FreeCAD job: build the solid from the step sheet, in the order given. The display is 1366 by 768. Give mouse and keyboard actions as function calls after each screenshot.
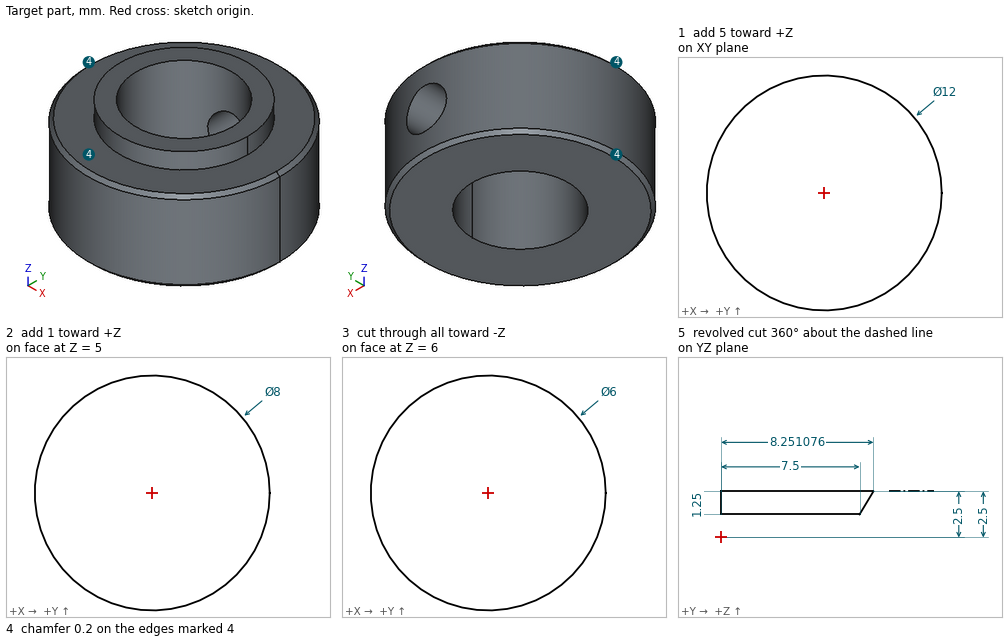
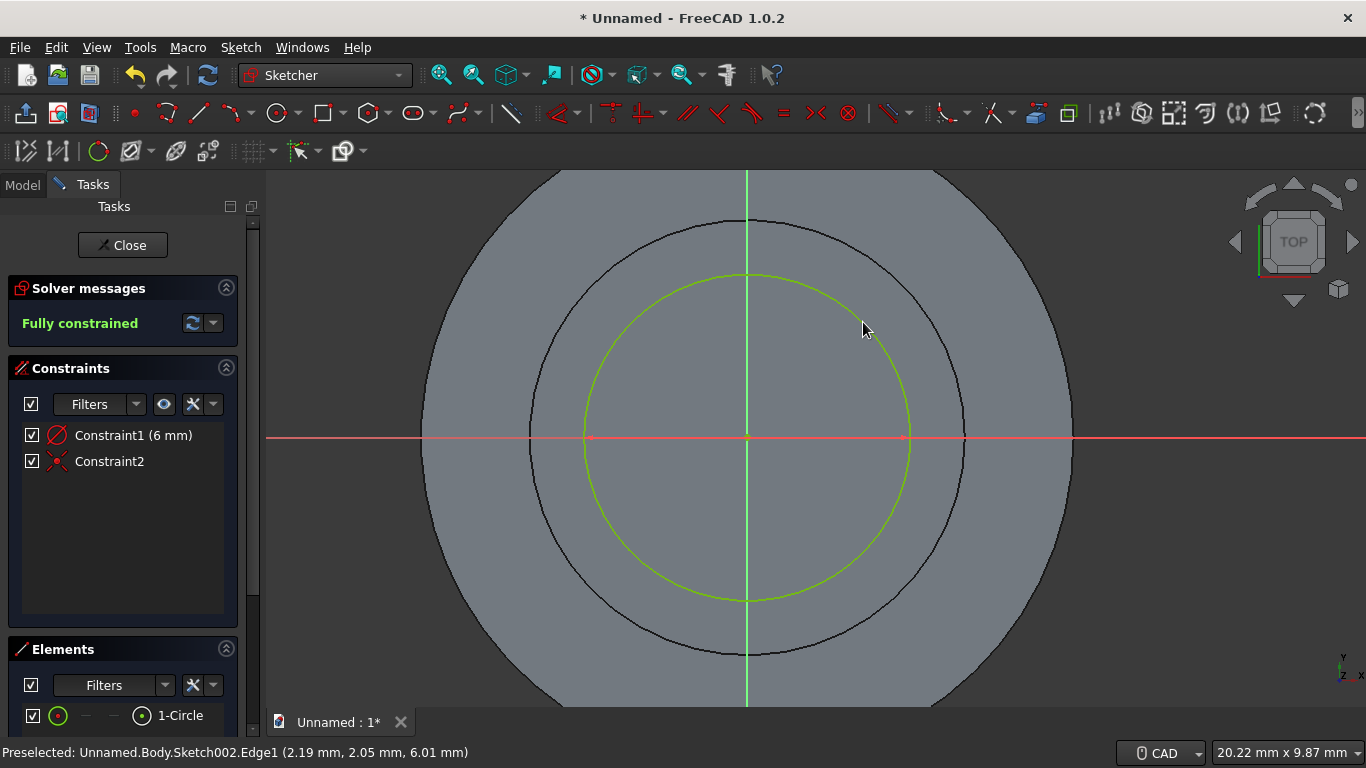
click(123, 245)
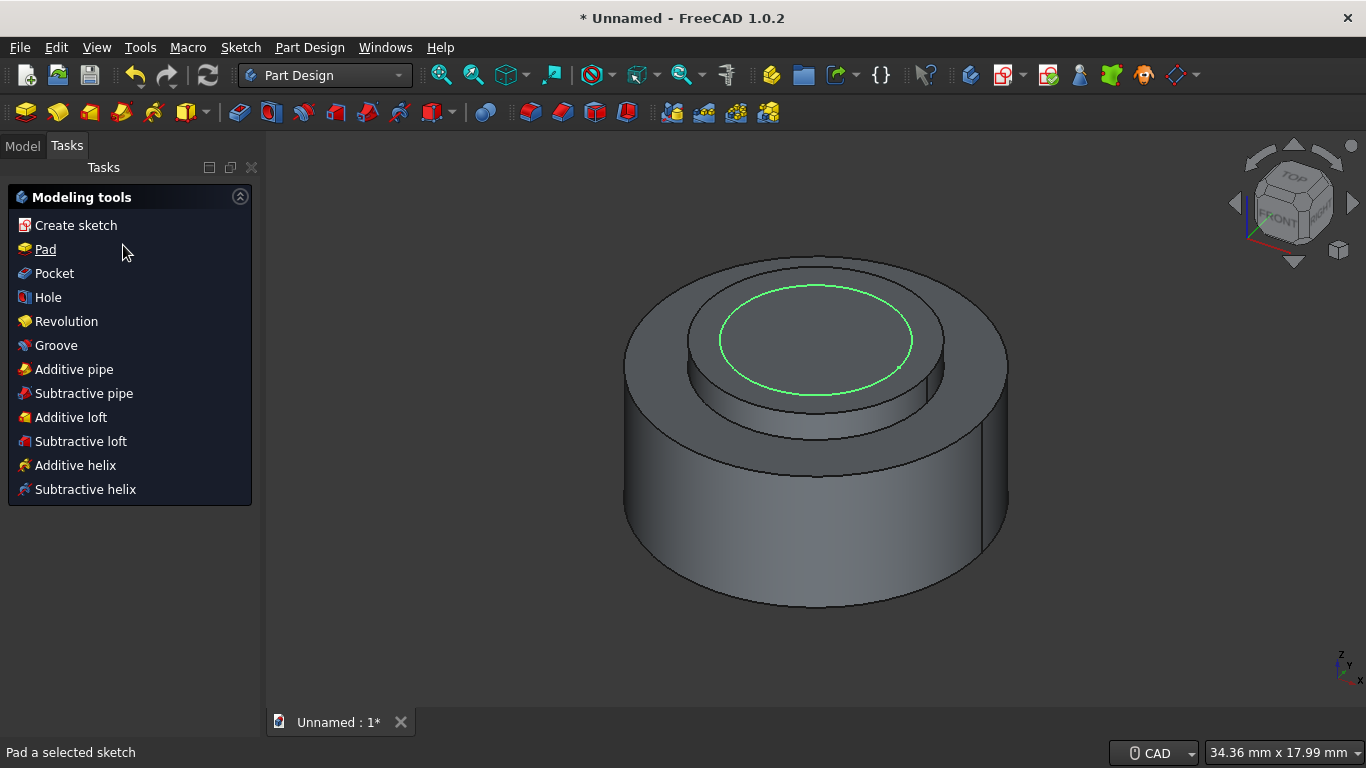
click(240, 112)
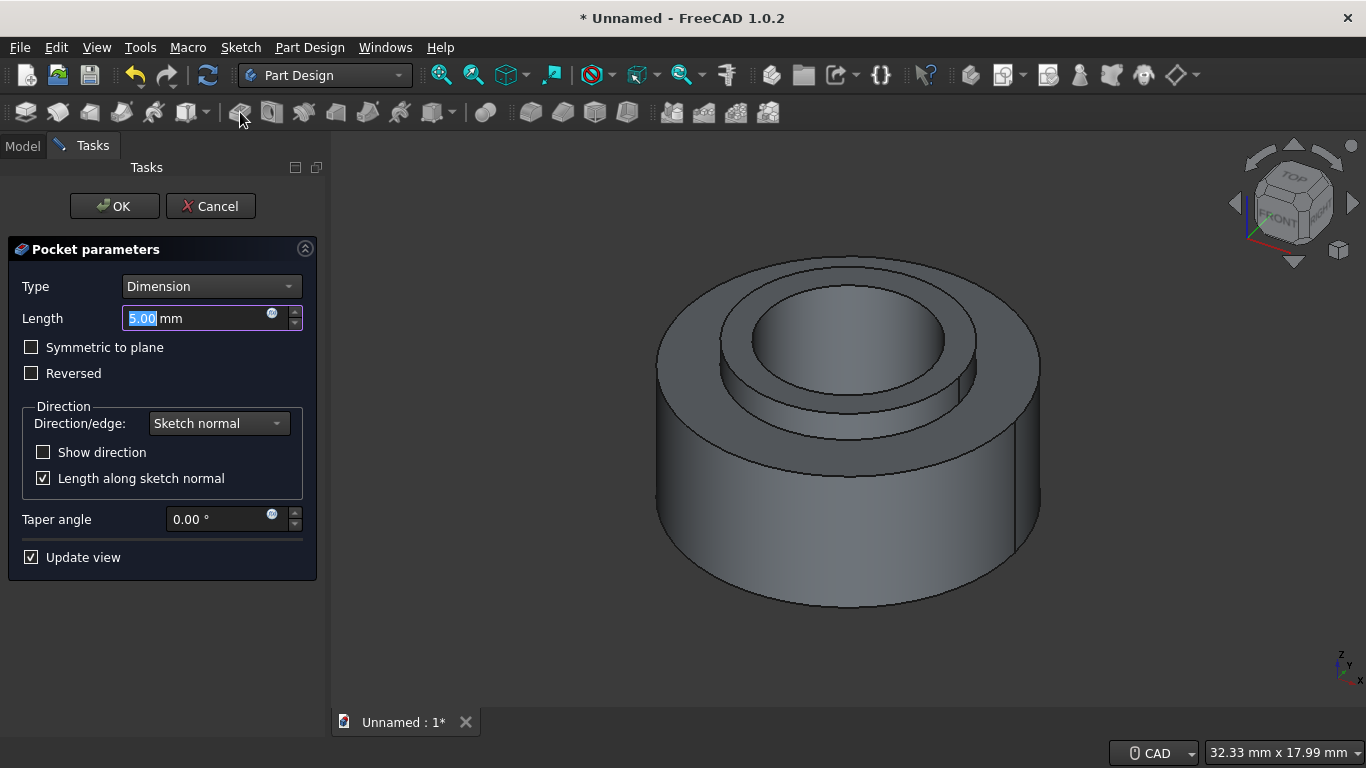
click(212, 286)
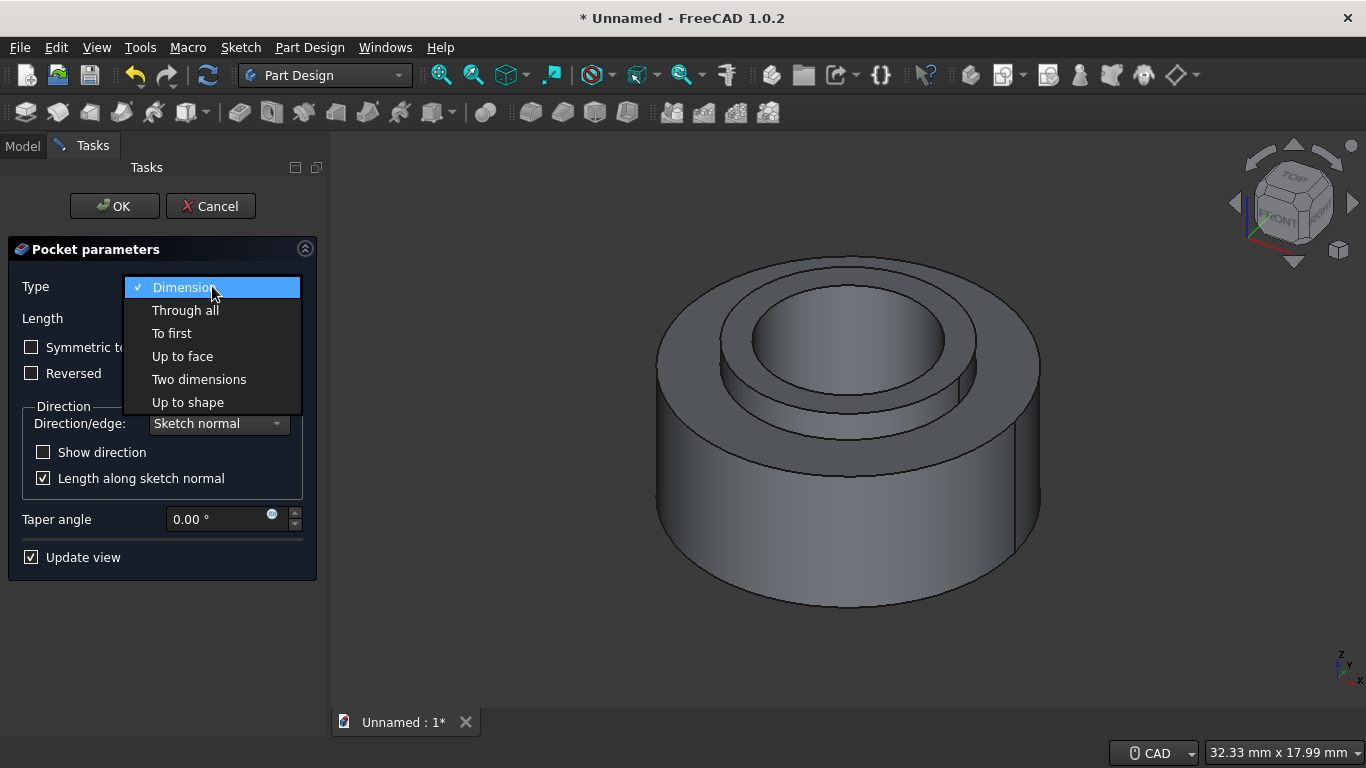
click(212, 310)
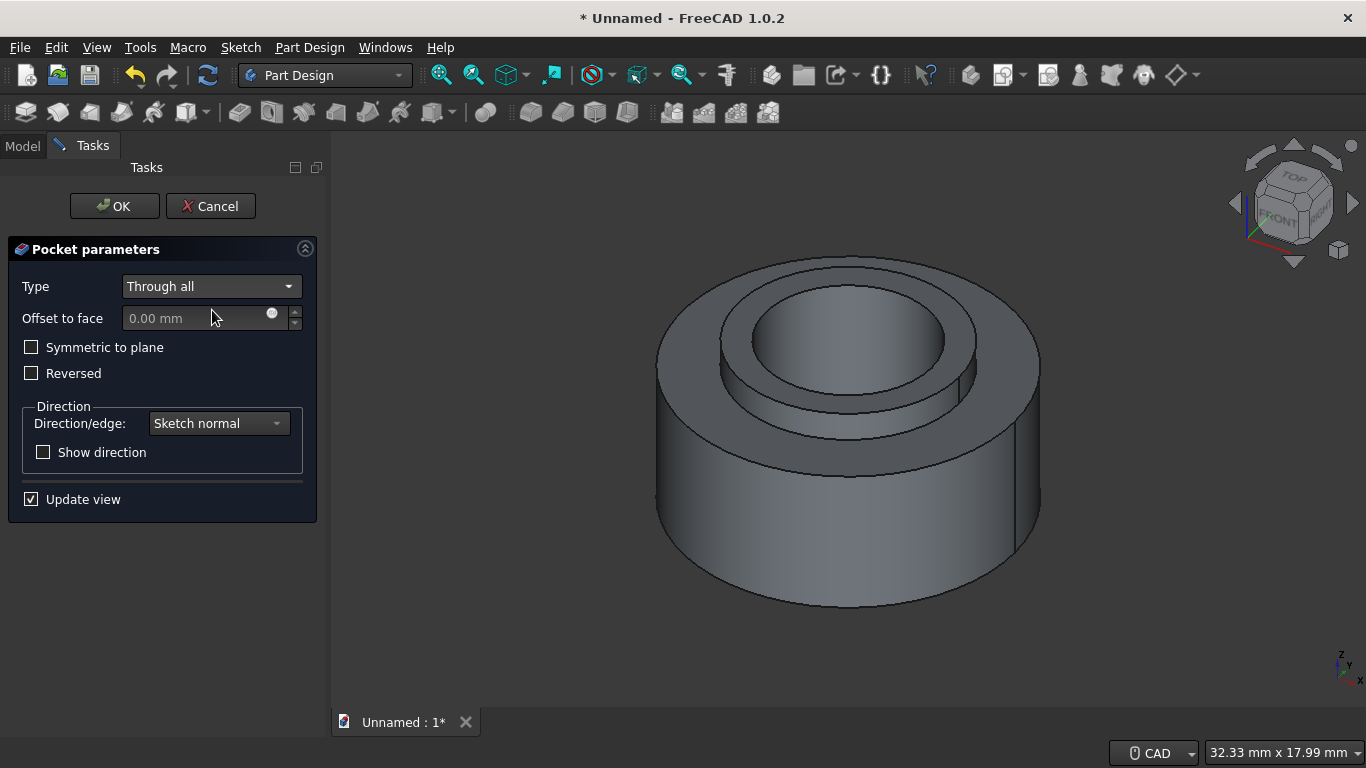
click(115, 206)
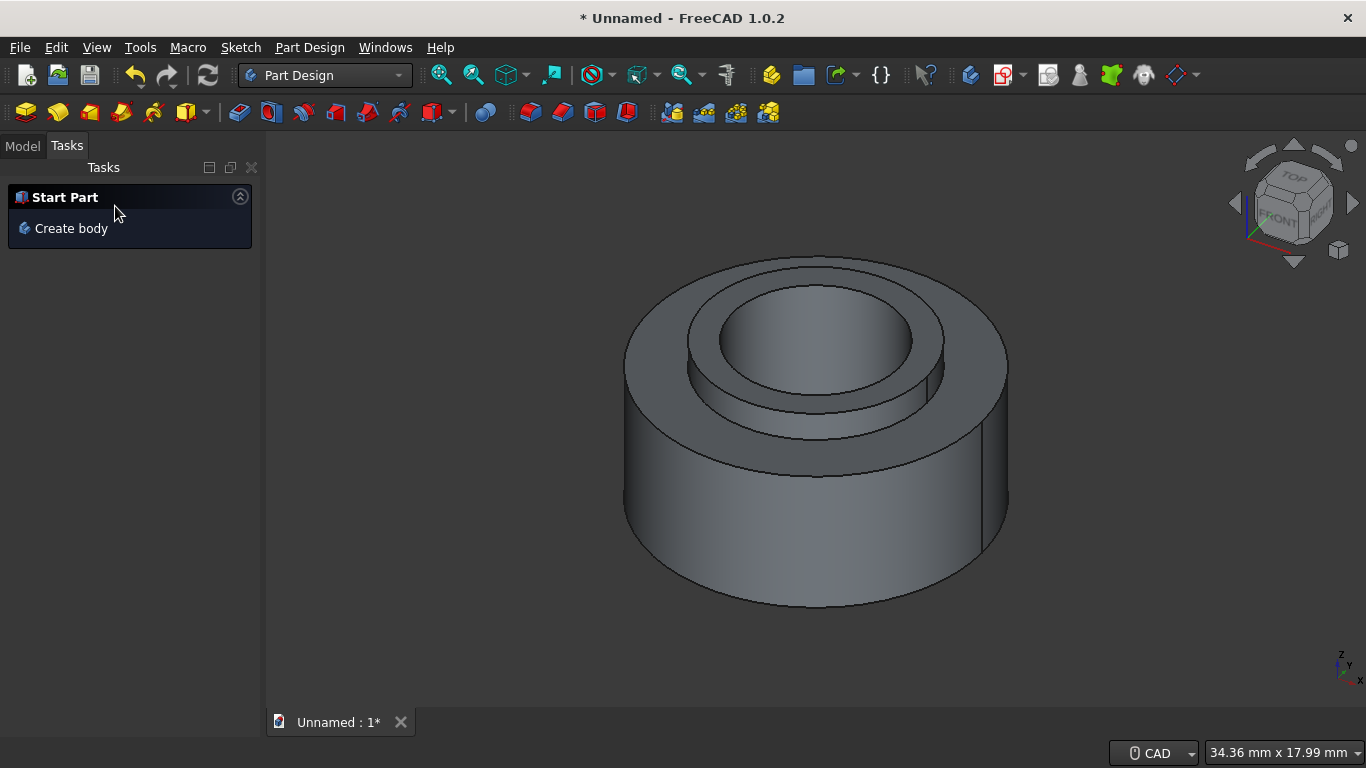
click(625, 377)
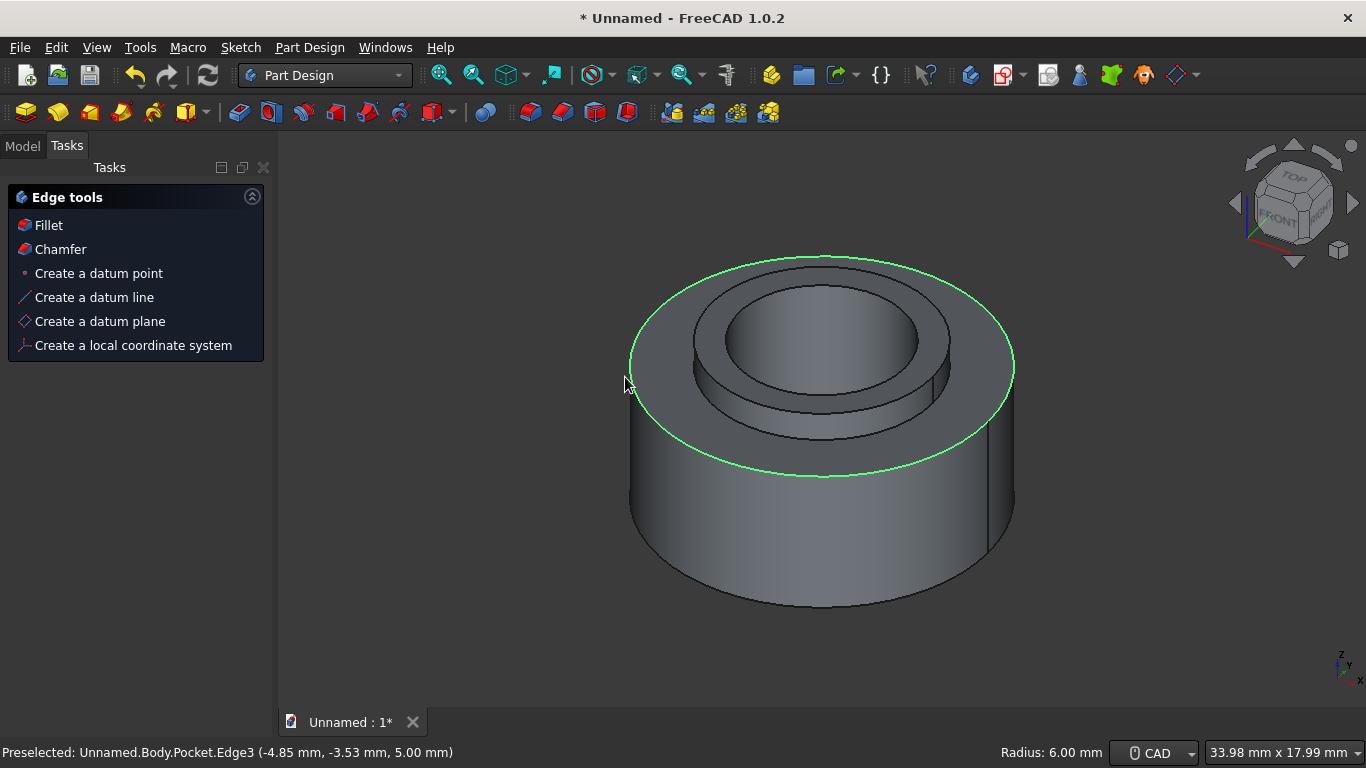
key(0)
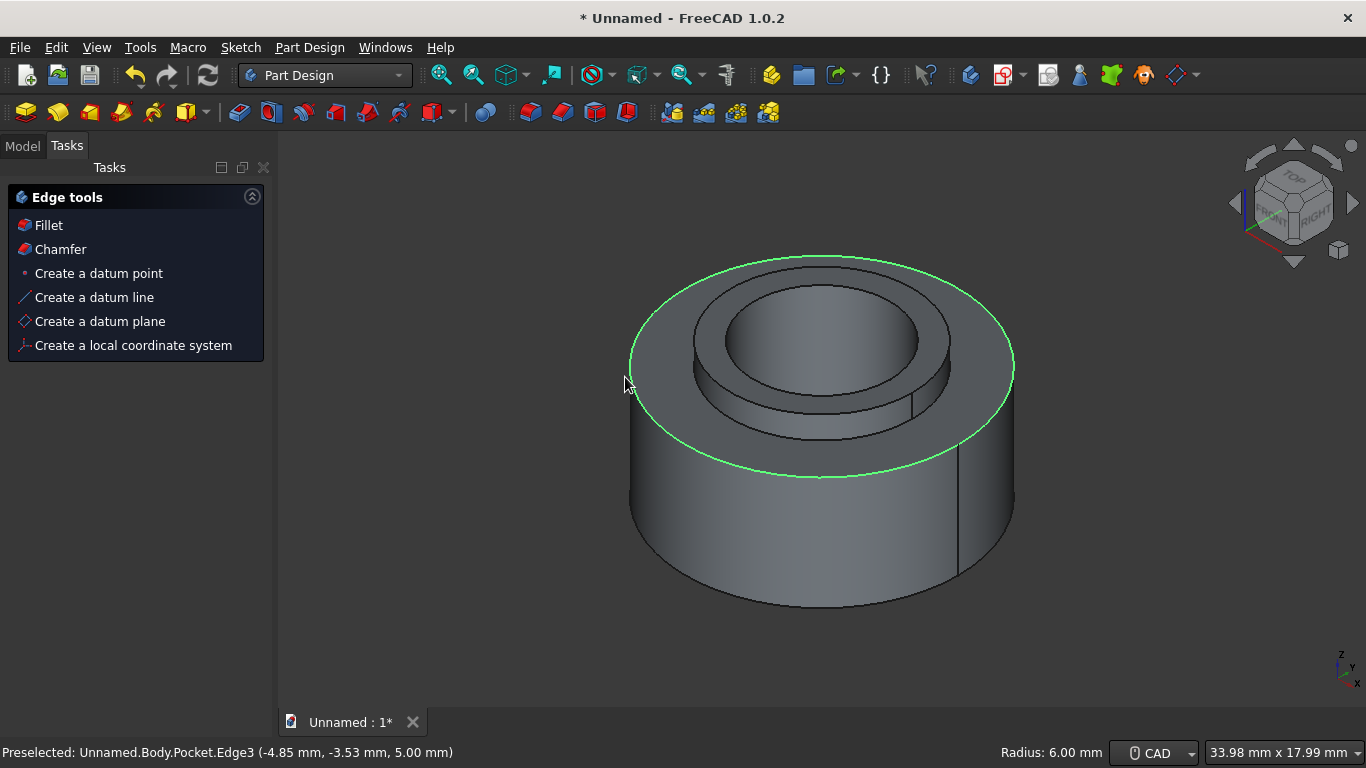
key(2)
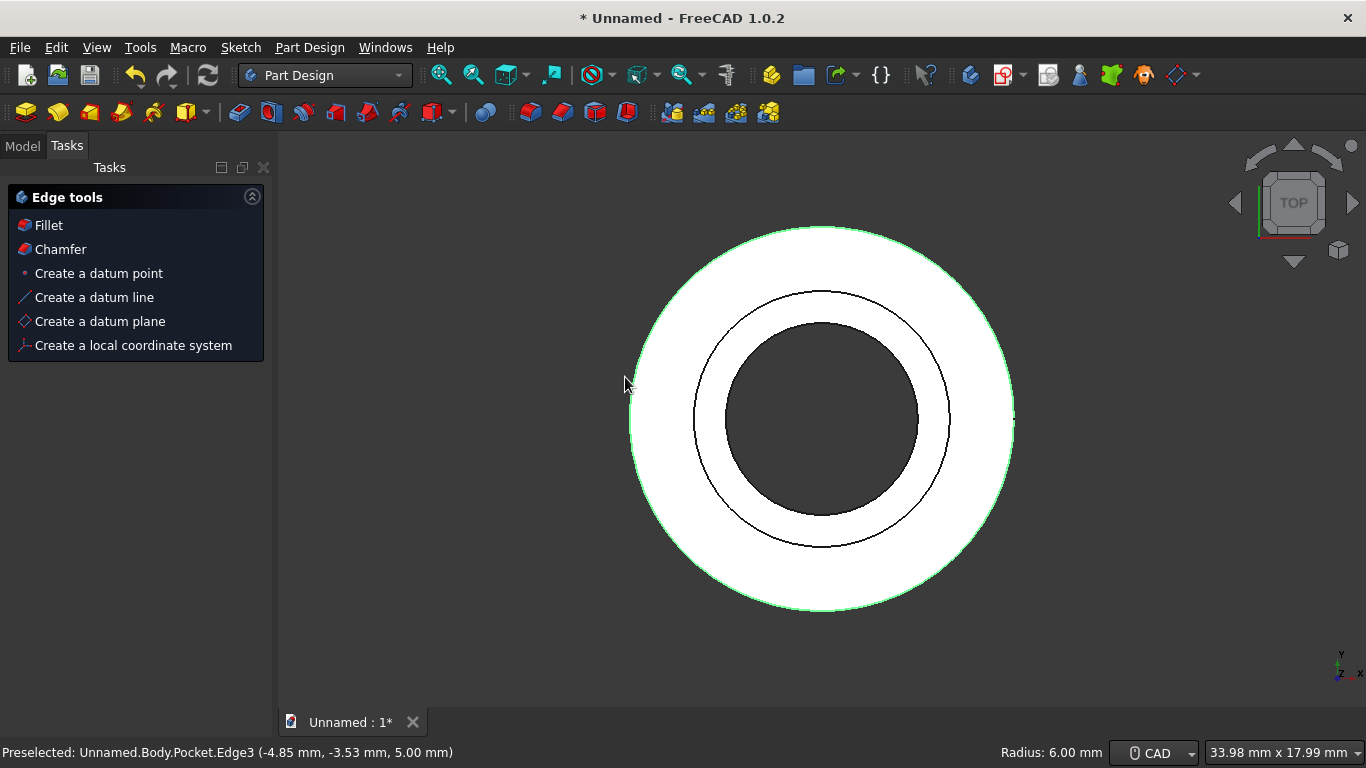
key(1)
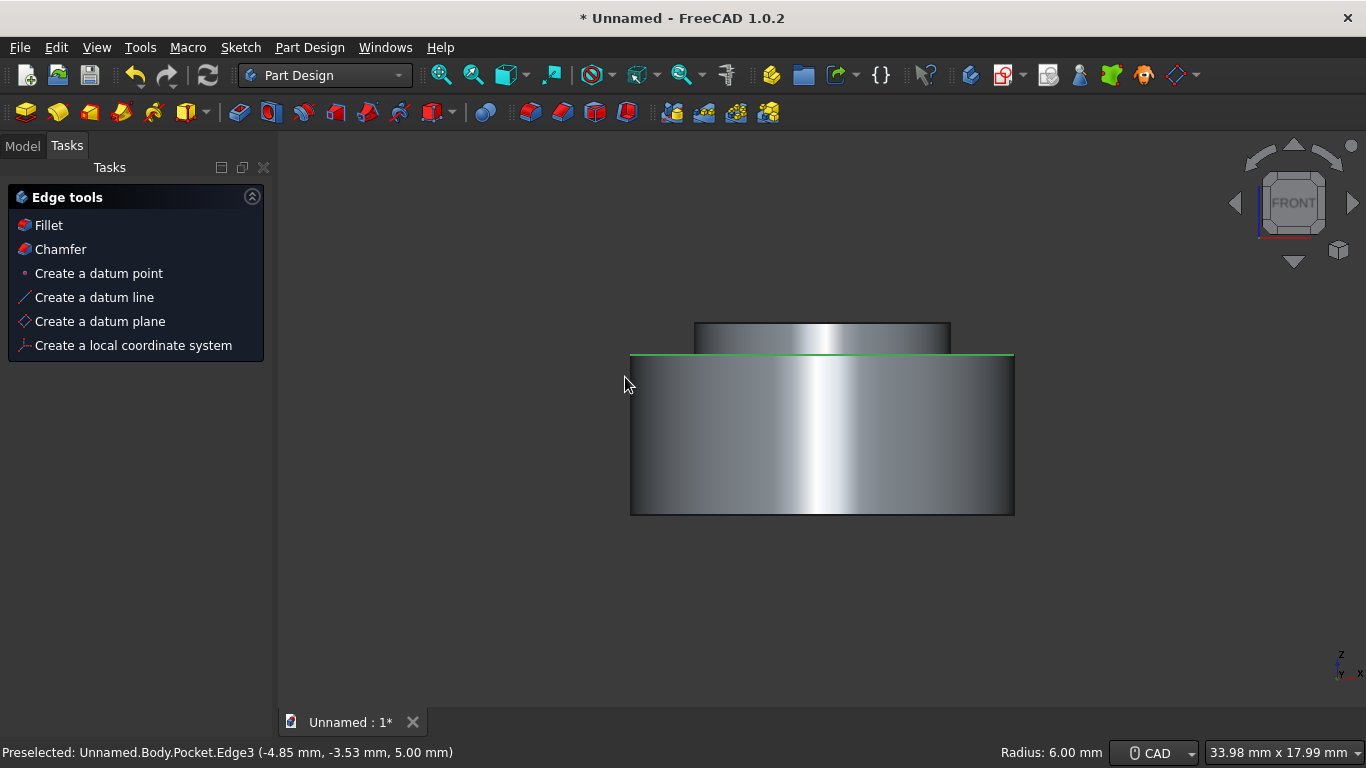
click(442, 76)